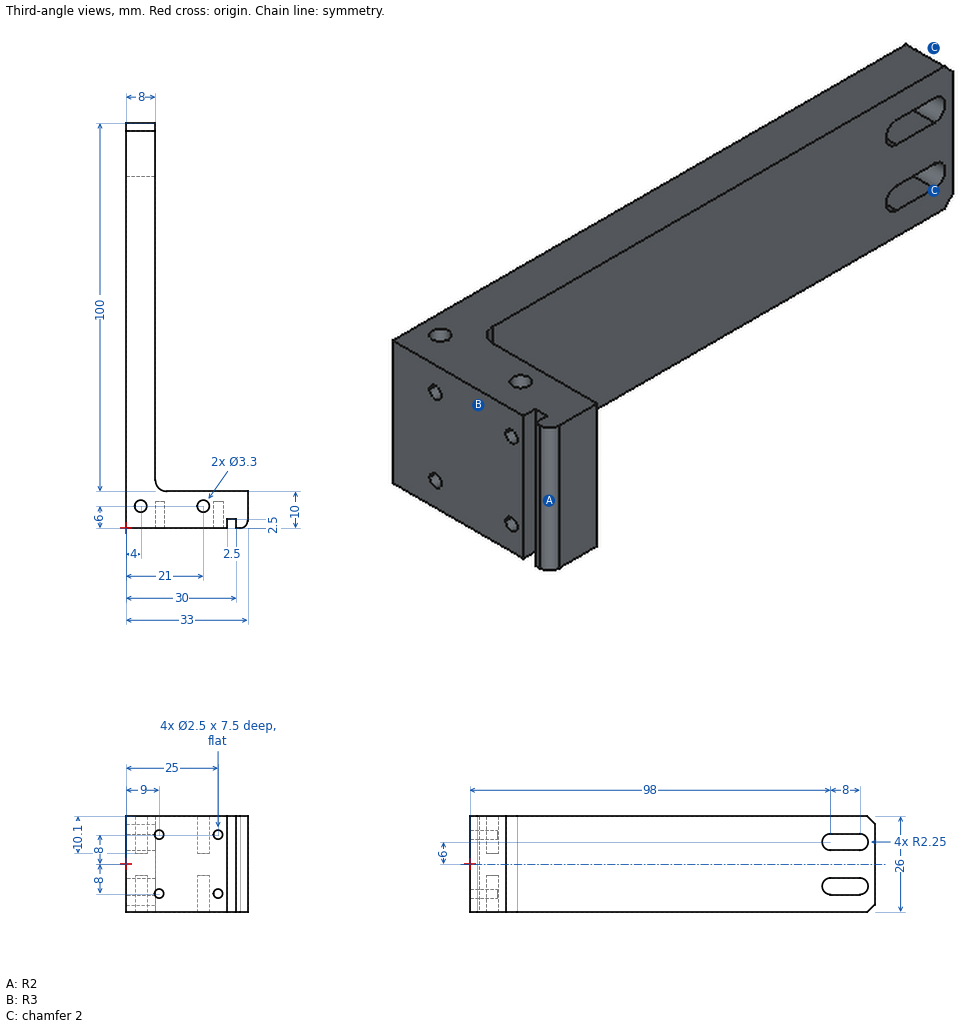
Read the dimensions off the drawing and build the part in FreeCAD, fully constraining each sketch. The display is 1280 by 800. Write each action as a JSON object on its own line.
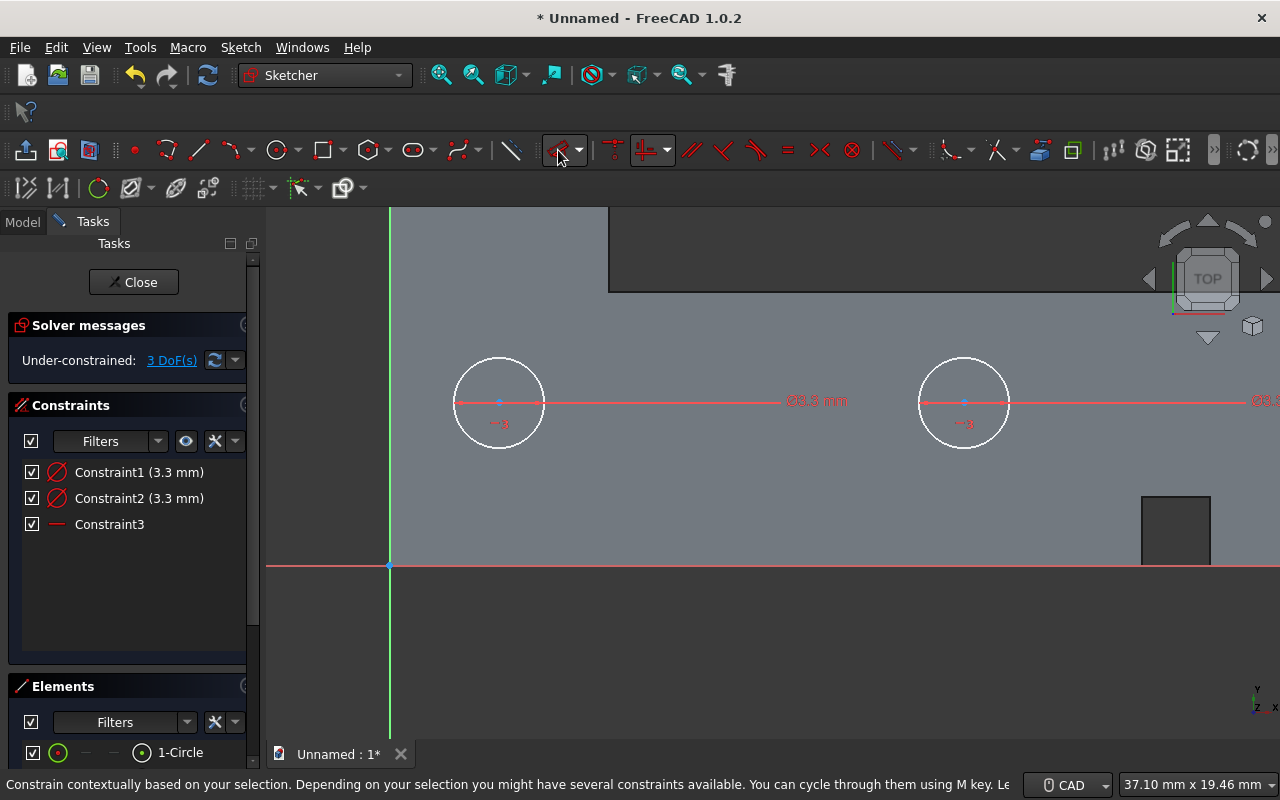
{"action": "left_click", "coordinate": [964, 403]}
{"action": "left_click", "coordinate": [356, 484]}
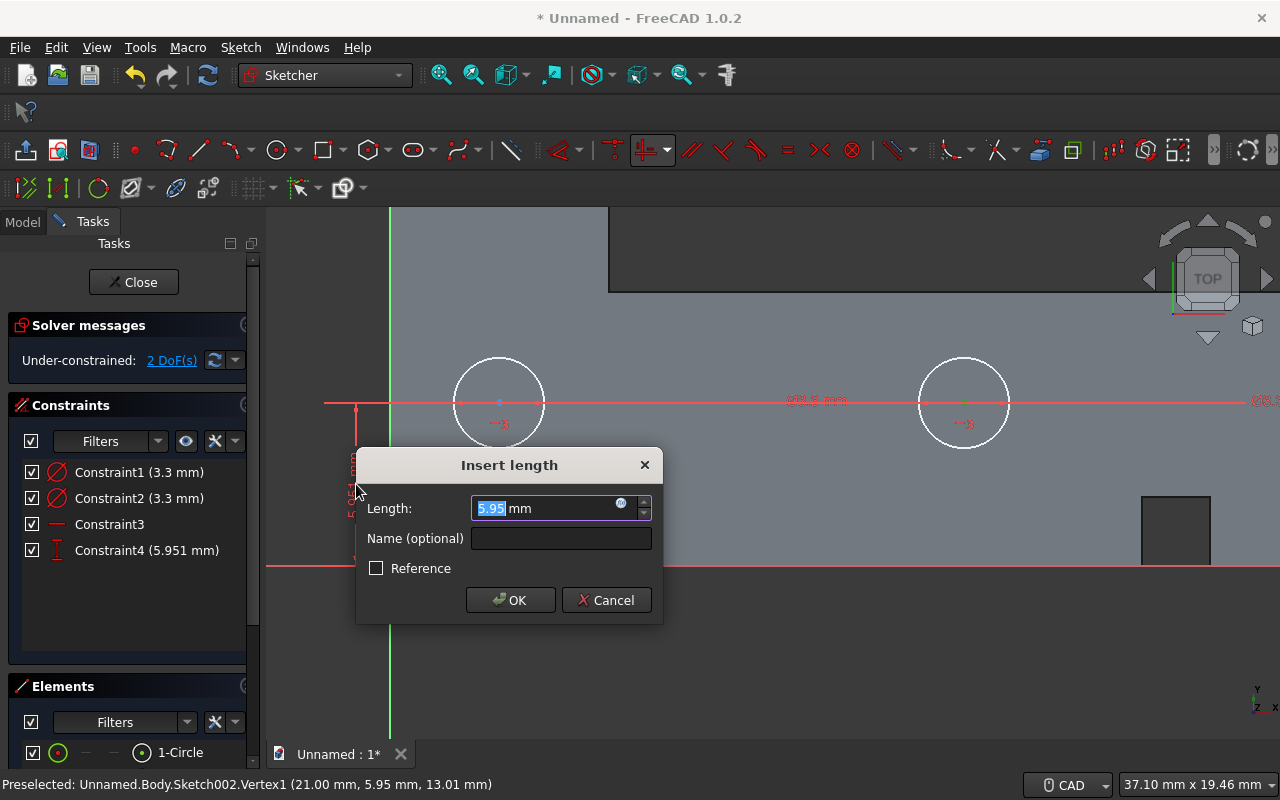
{"action": "type", "text": "6"}
{"action": "key", "text": "Return"}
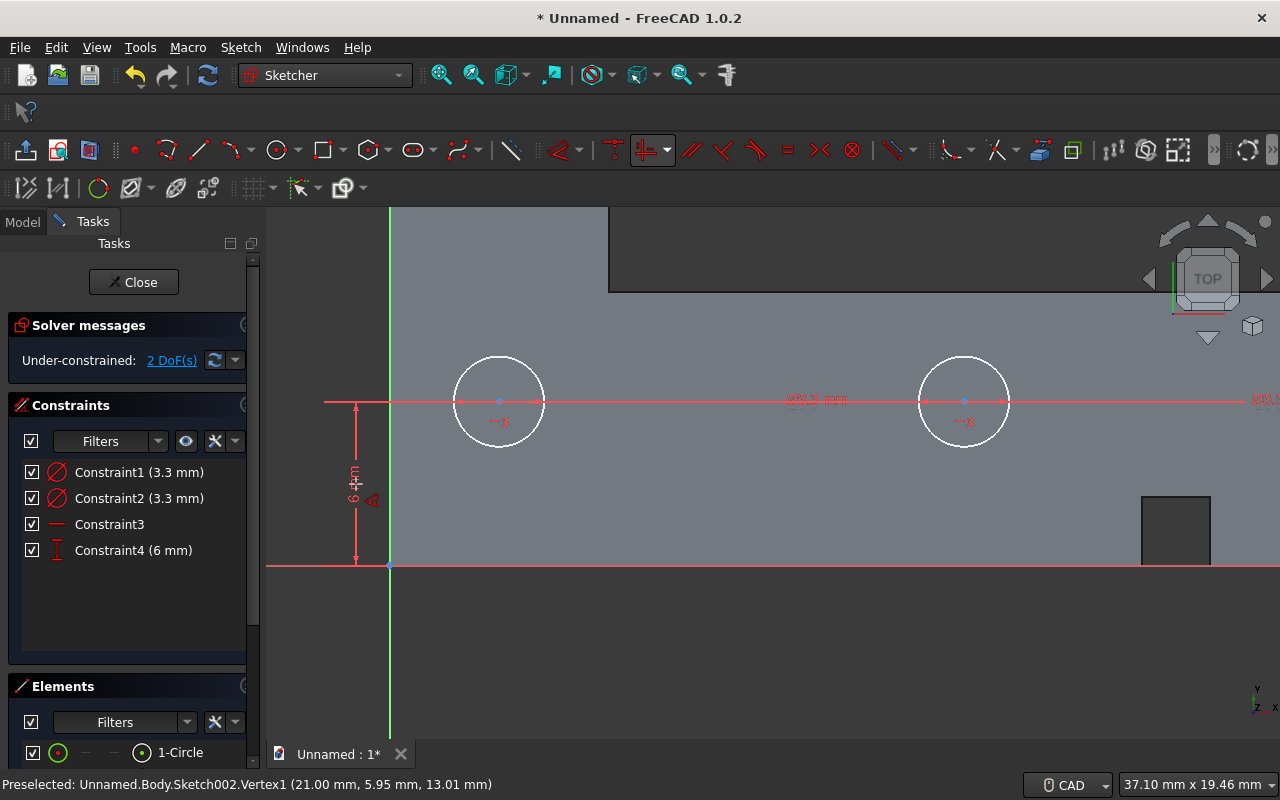
{"action": "left_click", "coordinate": [499, 402]}
{"action": "left_click", "coordinate": [444, 600]}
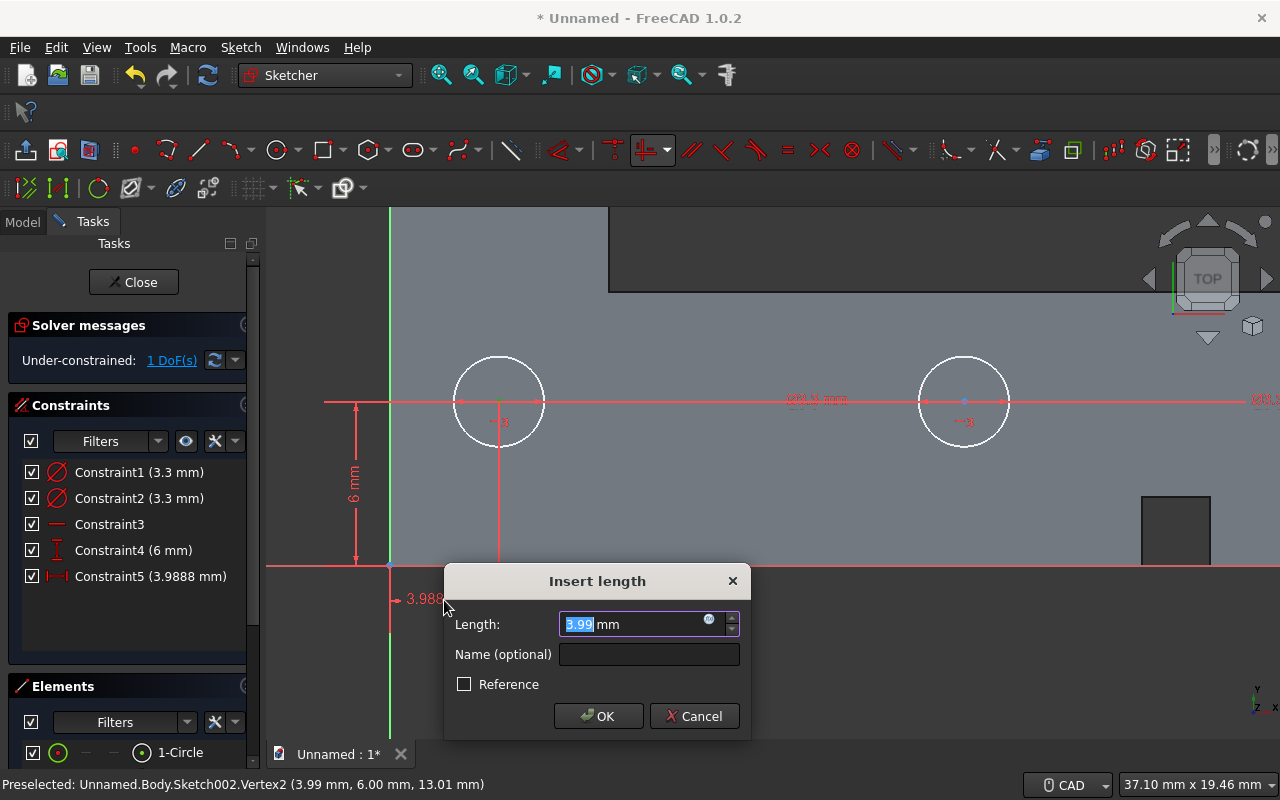
{"action": "type", "text": "4"}
{"action": "key", "text": "Return"}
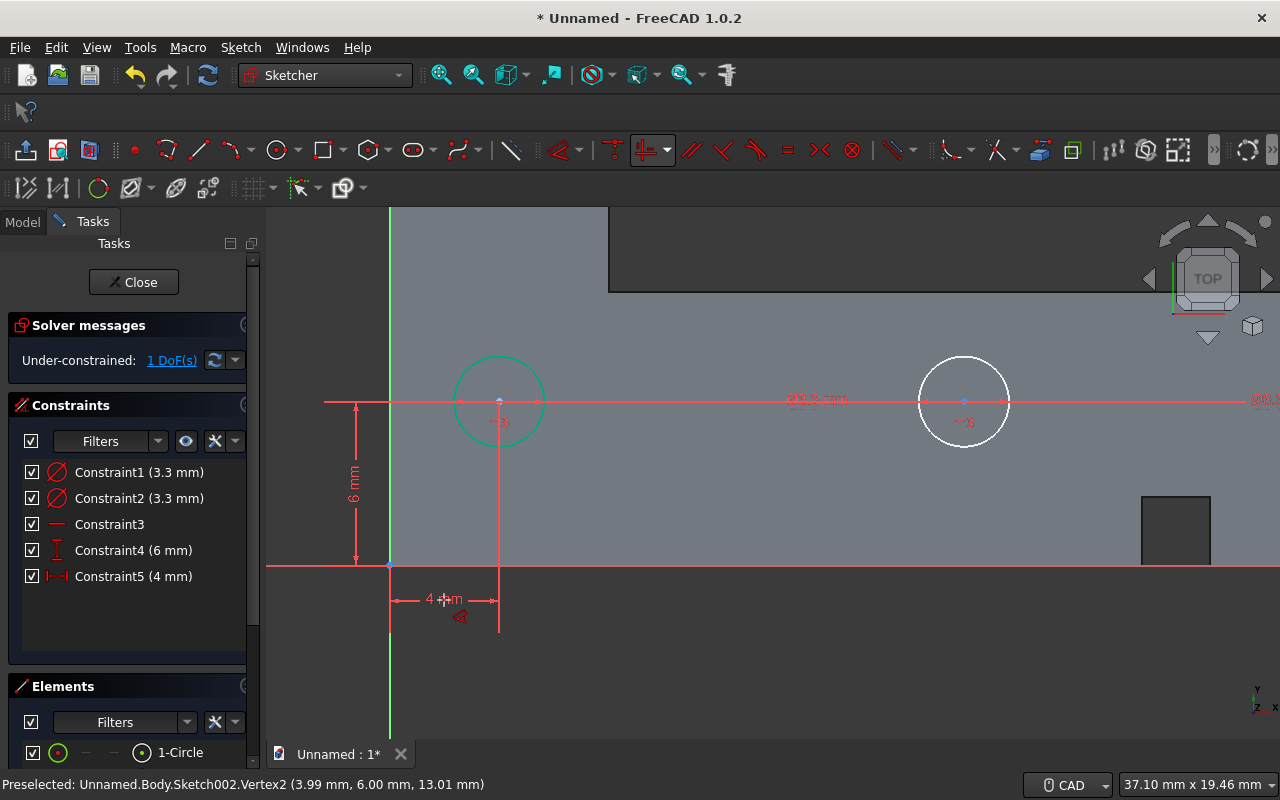
{"action": "left_click", "coordinate": [964, 402]}
{"action": "left_click", "coordinate": [677, 600]}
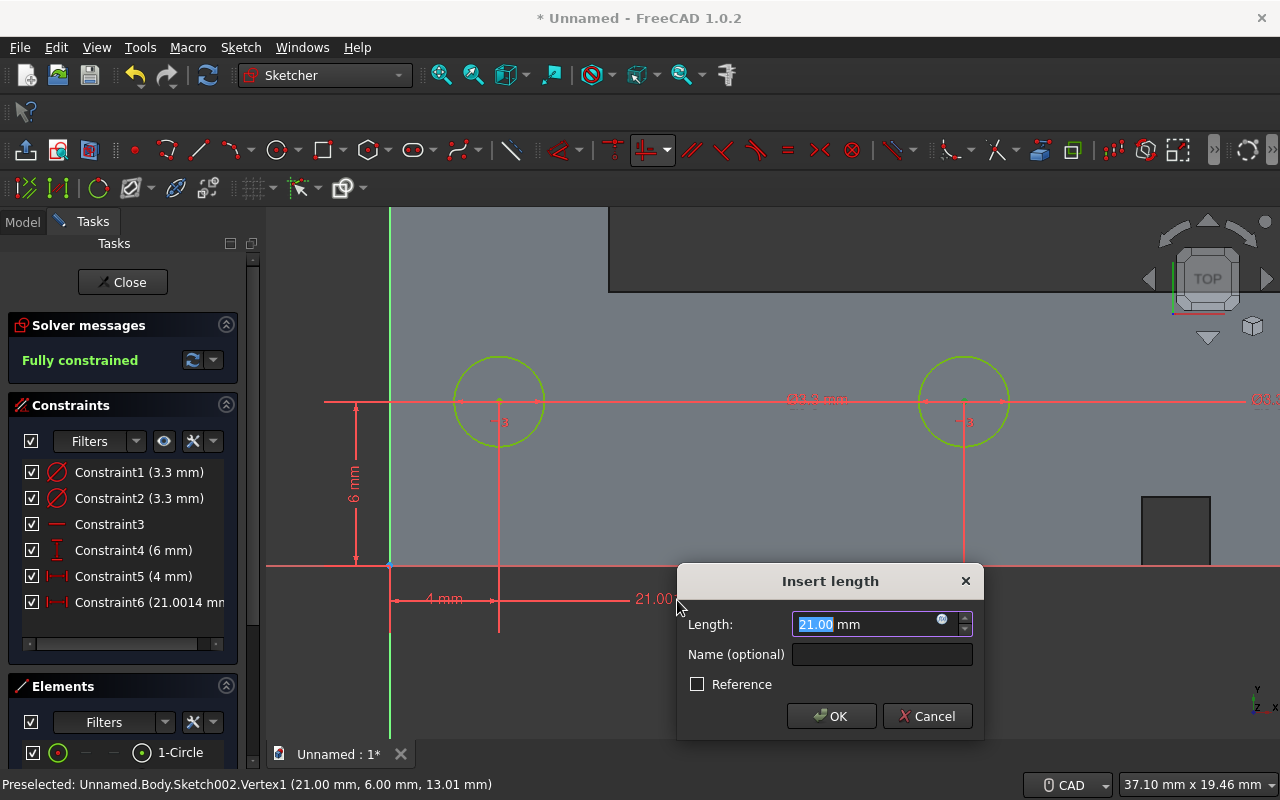
{"action": "type", "text": "21"}
{"action": "key", "text": "Return"}
{"action": "key", "text": "Escape"}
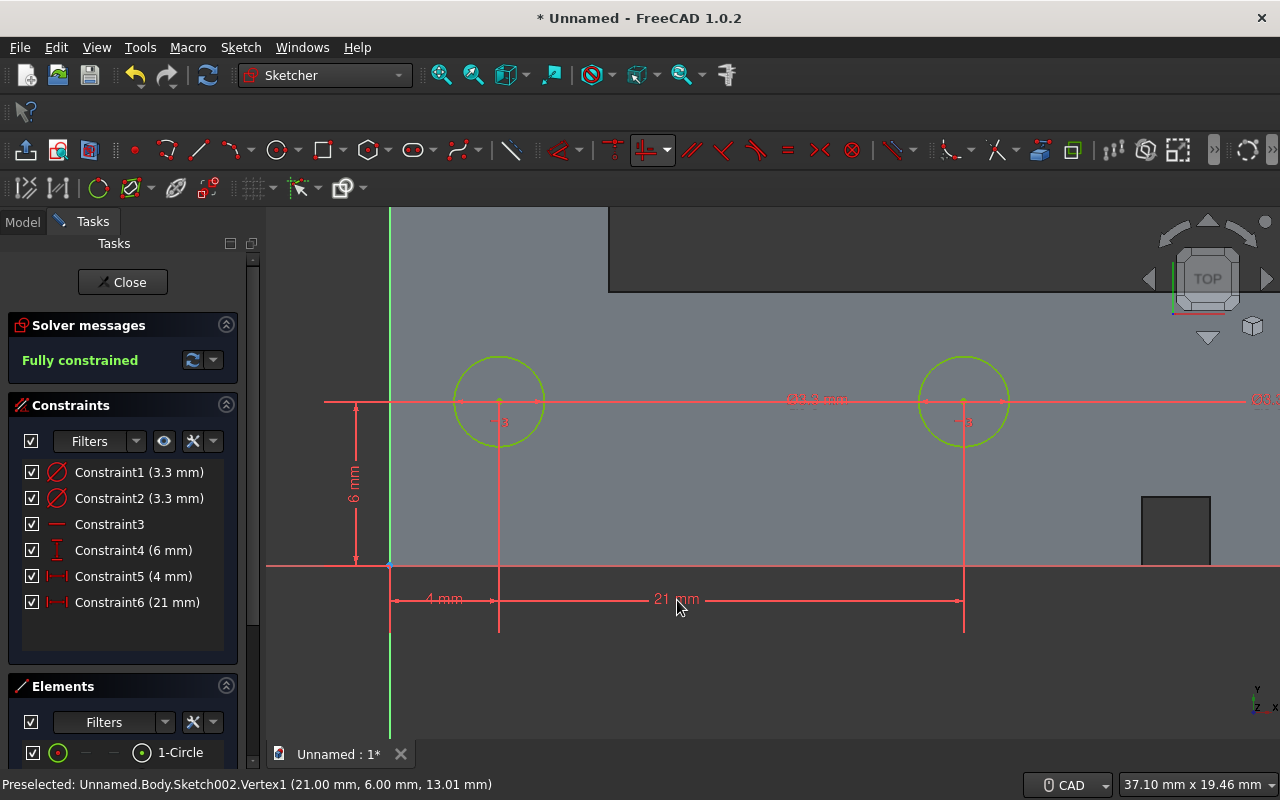
{"action": "left_click", "coordinate": [123, 282]}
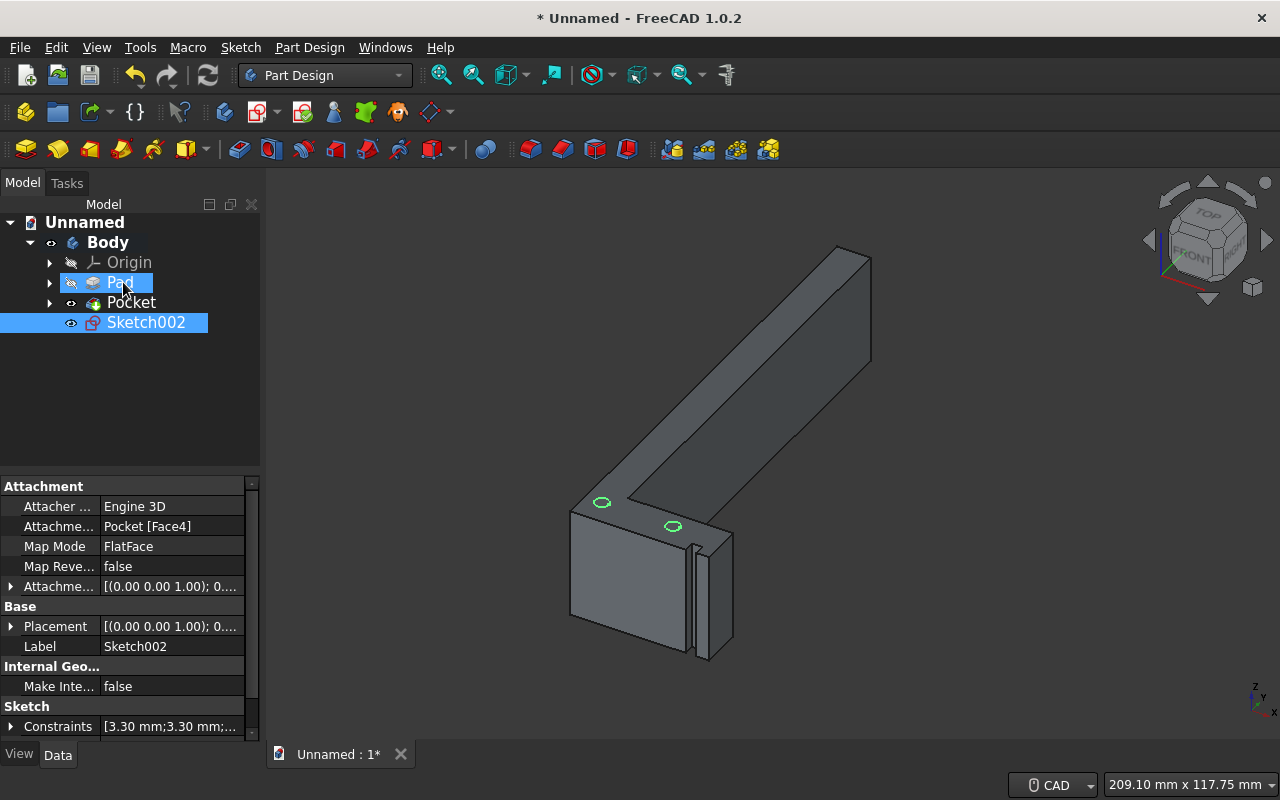
{"action": "left_click", "coordinate": [240, 150]}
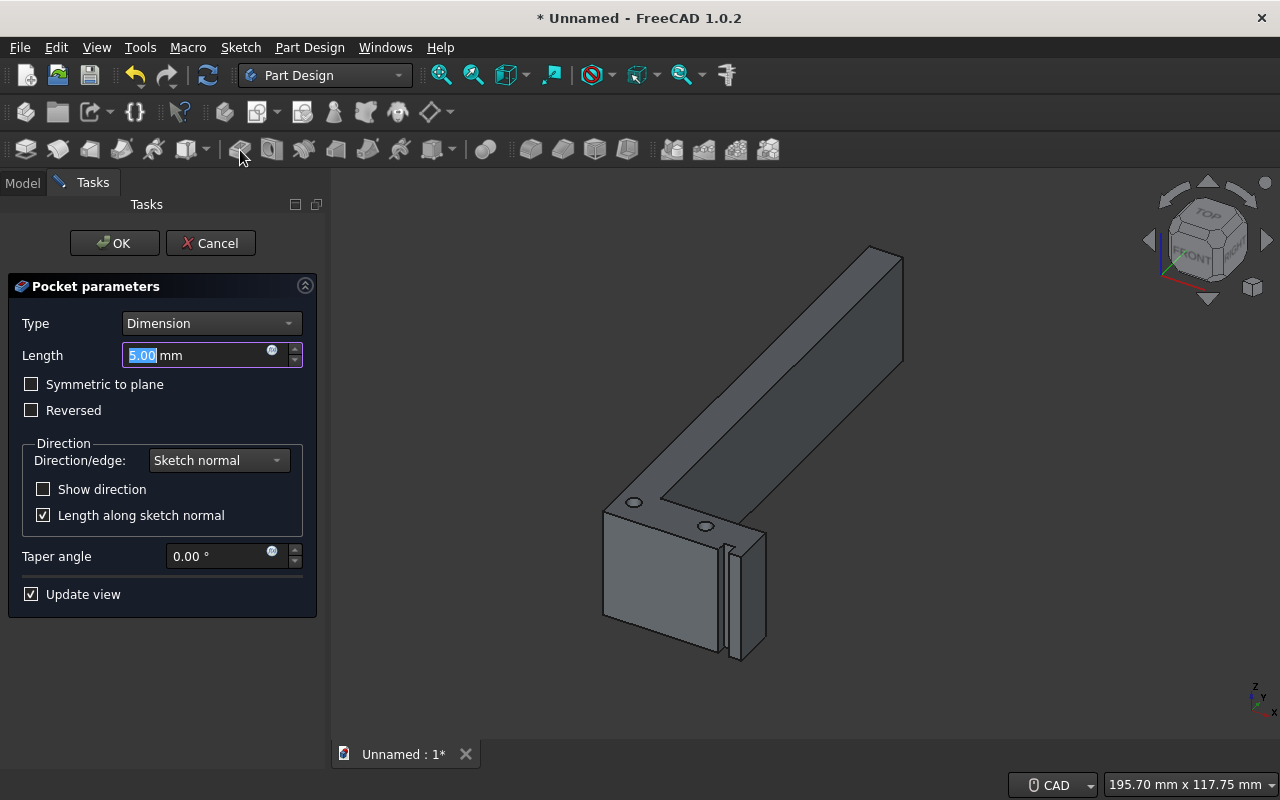
{"action": "type", "text": "10.1"}
{"action": "key", "text": "Tab"}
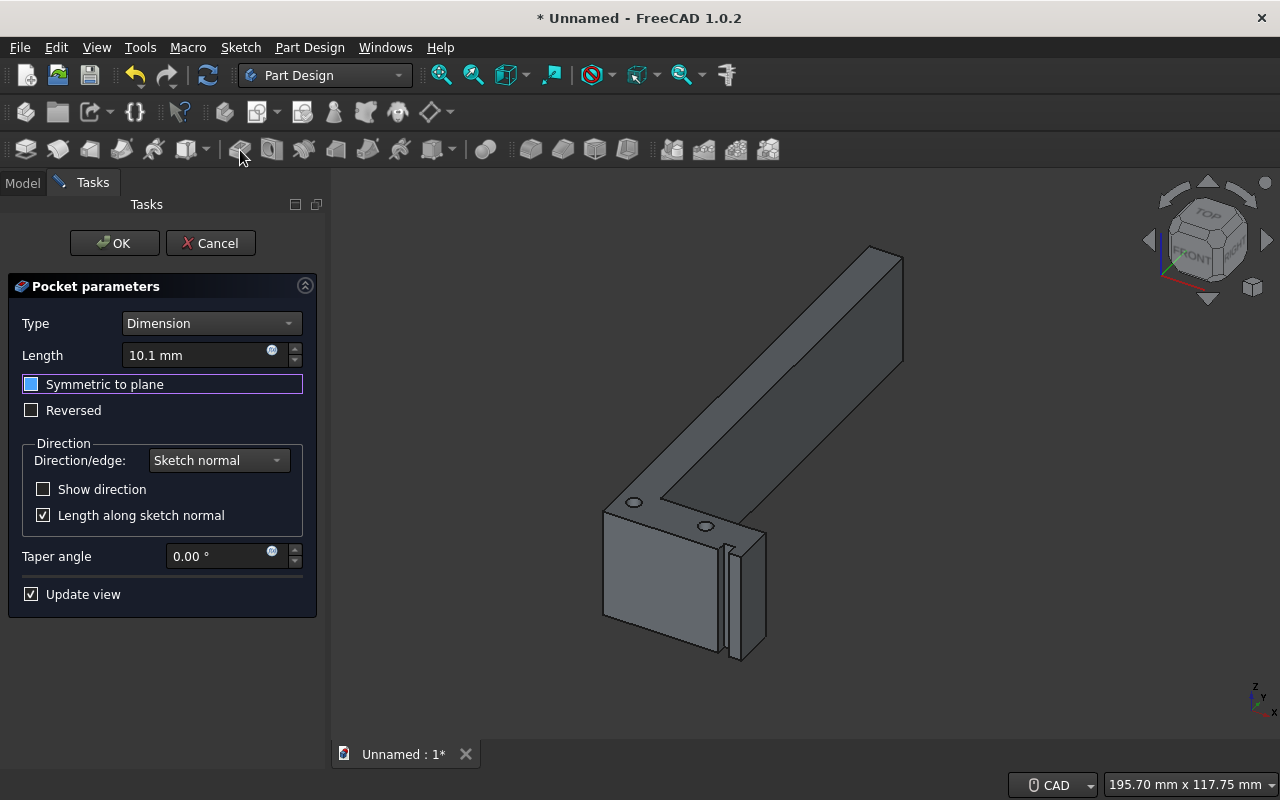
{"action": "left_click", "coordinate": [115, 243]}